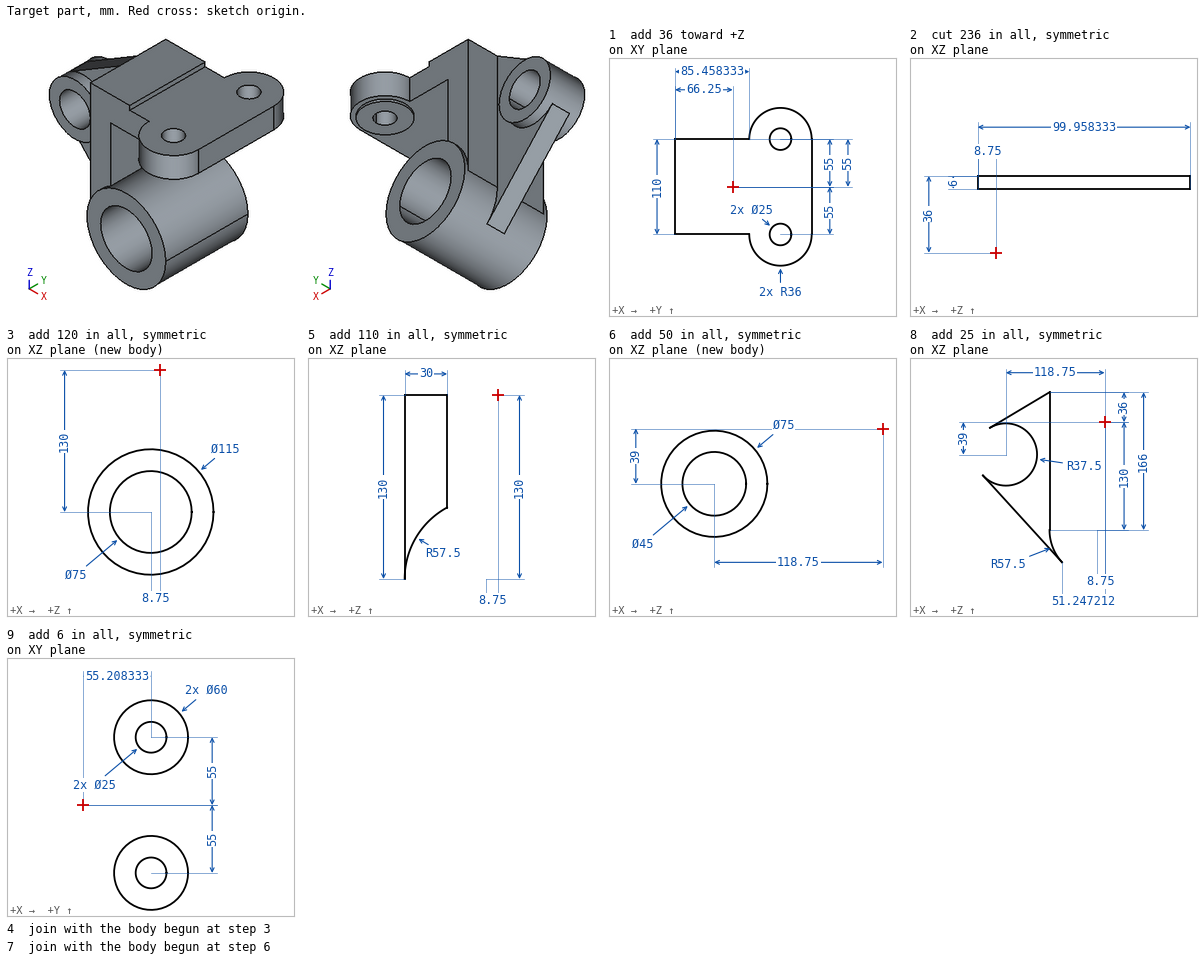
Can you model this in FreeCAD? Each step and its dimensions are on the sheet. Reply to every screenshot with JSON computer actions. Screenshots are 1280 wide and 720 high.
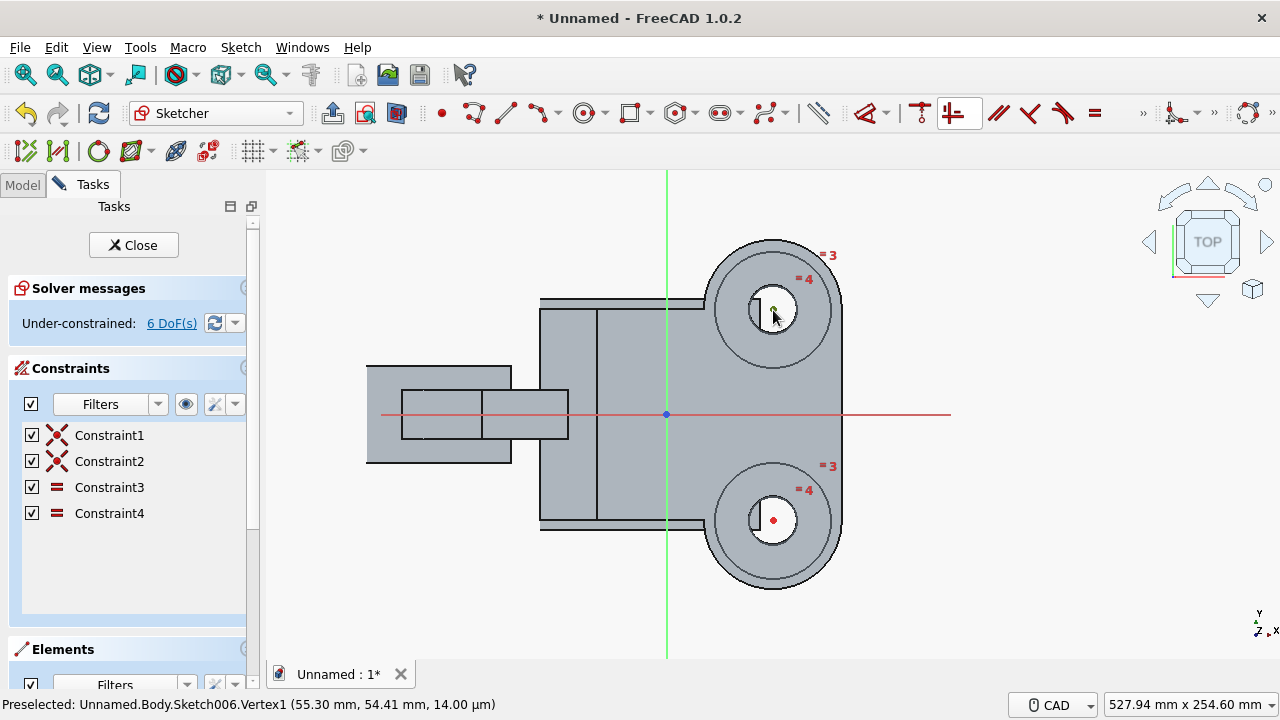
{"action": "left_click", "coordinate": [773, 521]}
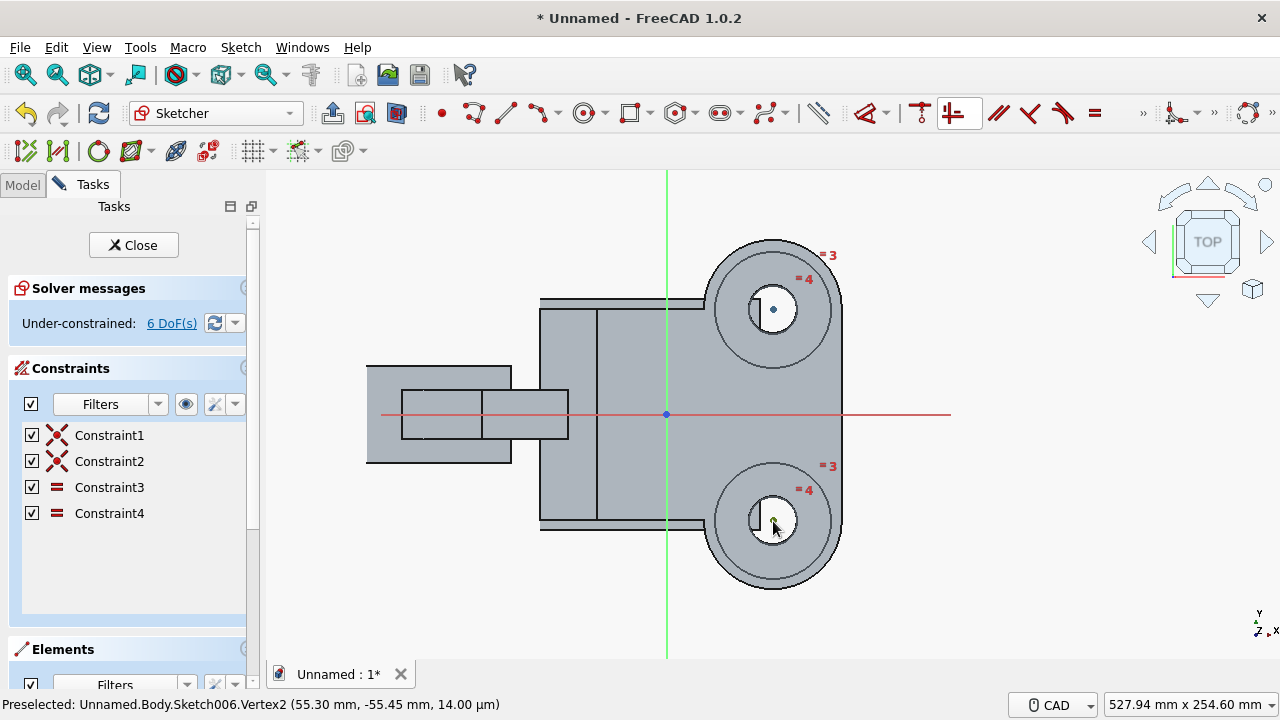
{"action": "key", "text": "v"}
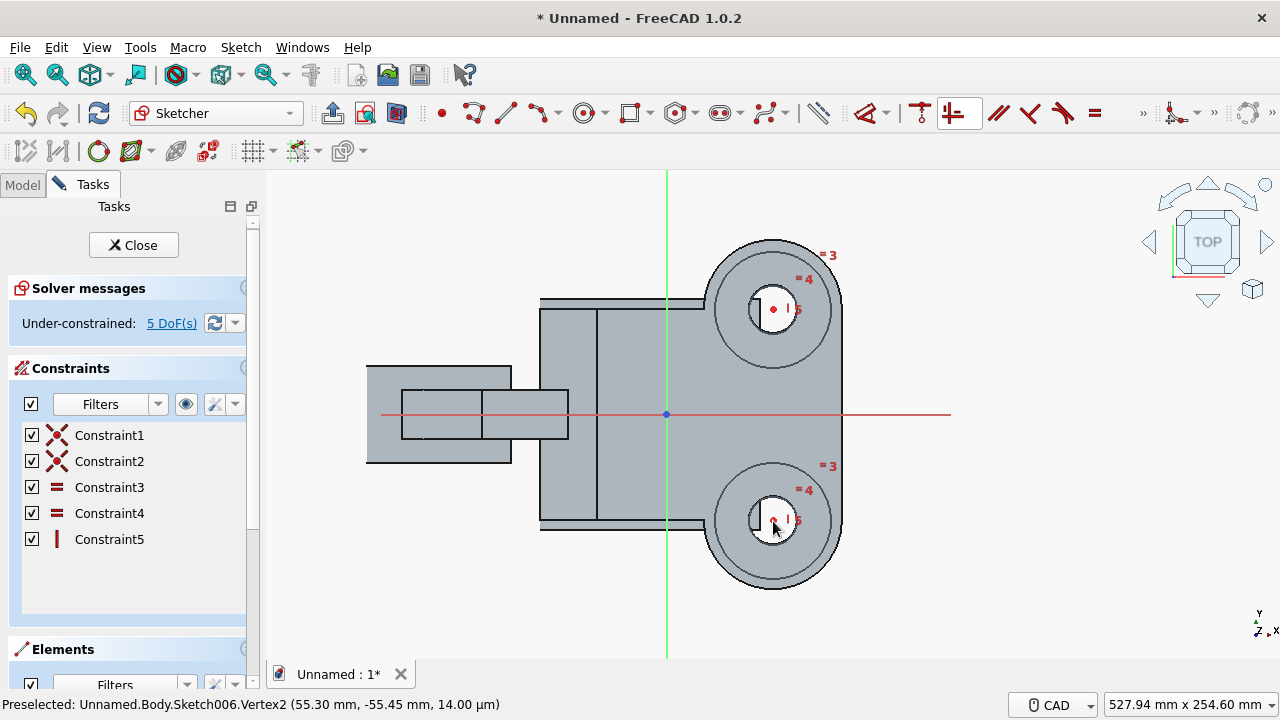
{"action": "left_click", "coordinate": [866, 114]}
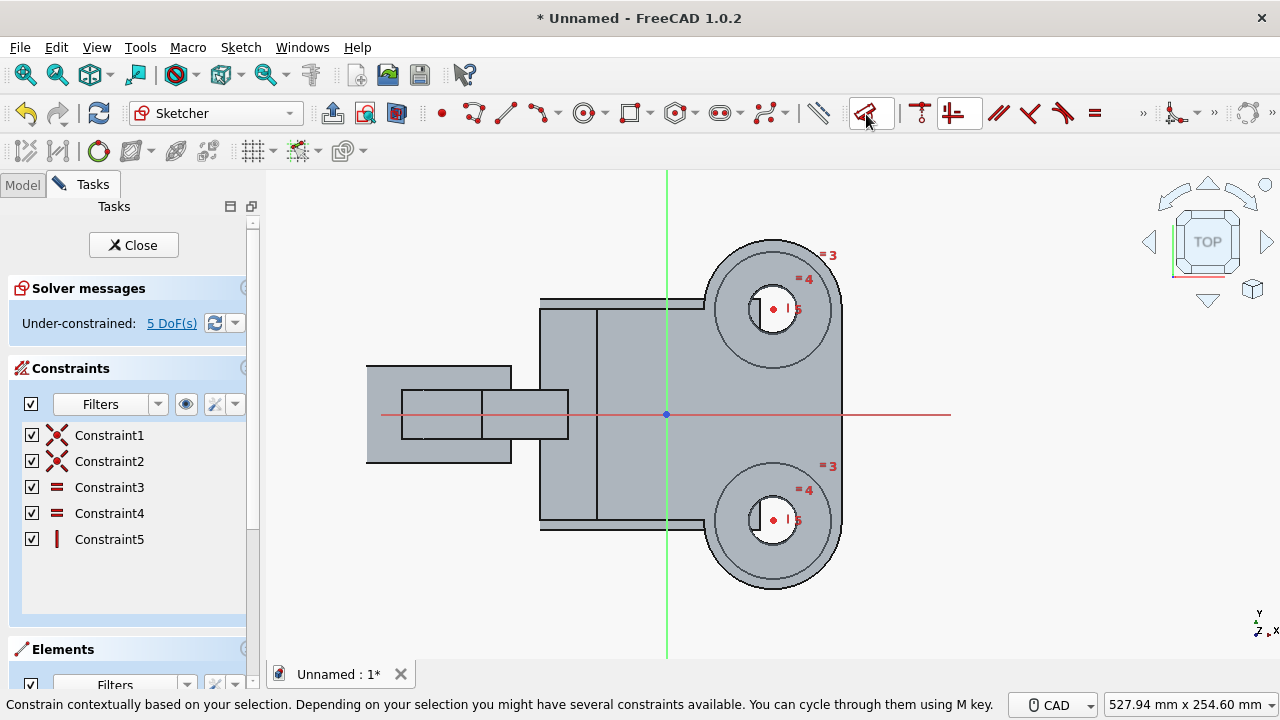
{"action": "left_click", "coordinate": [814, 269]}
{"action": "left_click", "coordinate": [837, 246]}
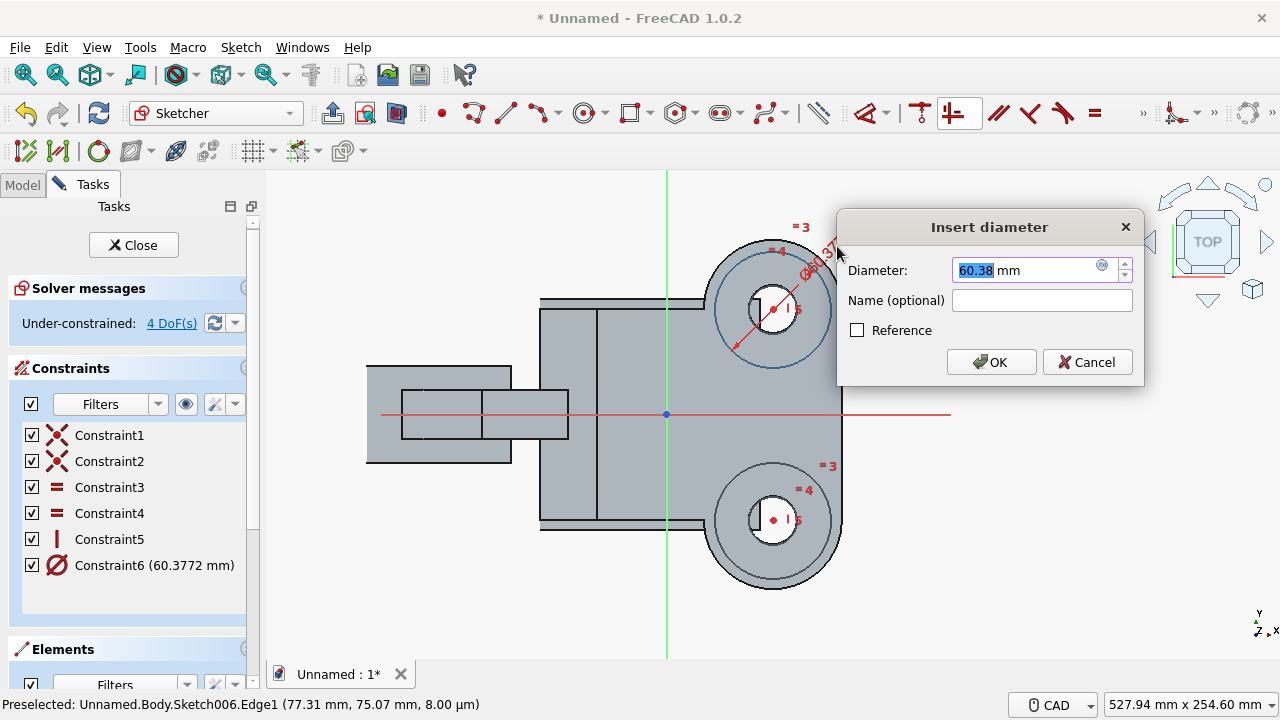
{"action": "type", "text": "60"}
{"action": "key", "text": "Return"}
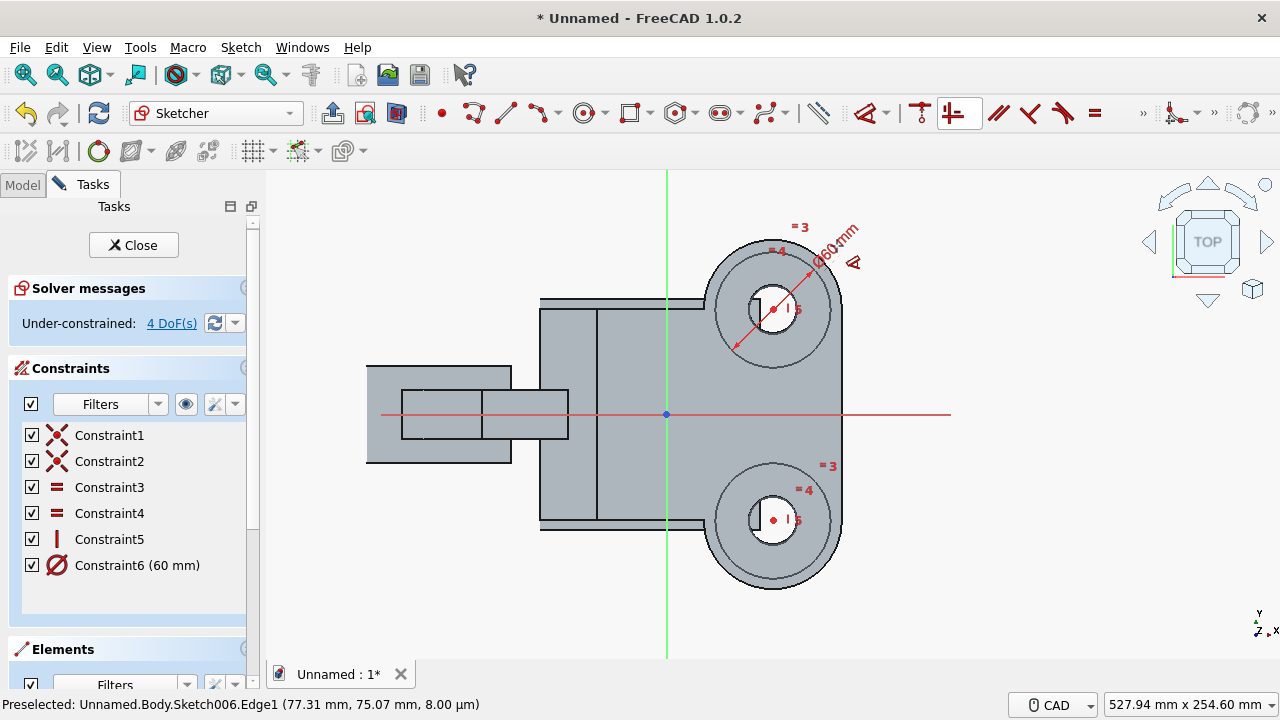
{"action": "left_click", "coordinate": [790, 293]}
{"action": "left_click", "coordinate": [849, 288]}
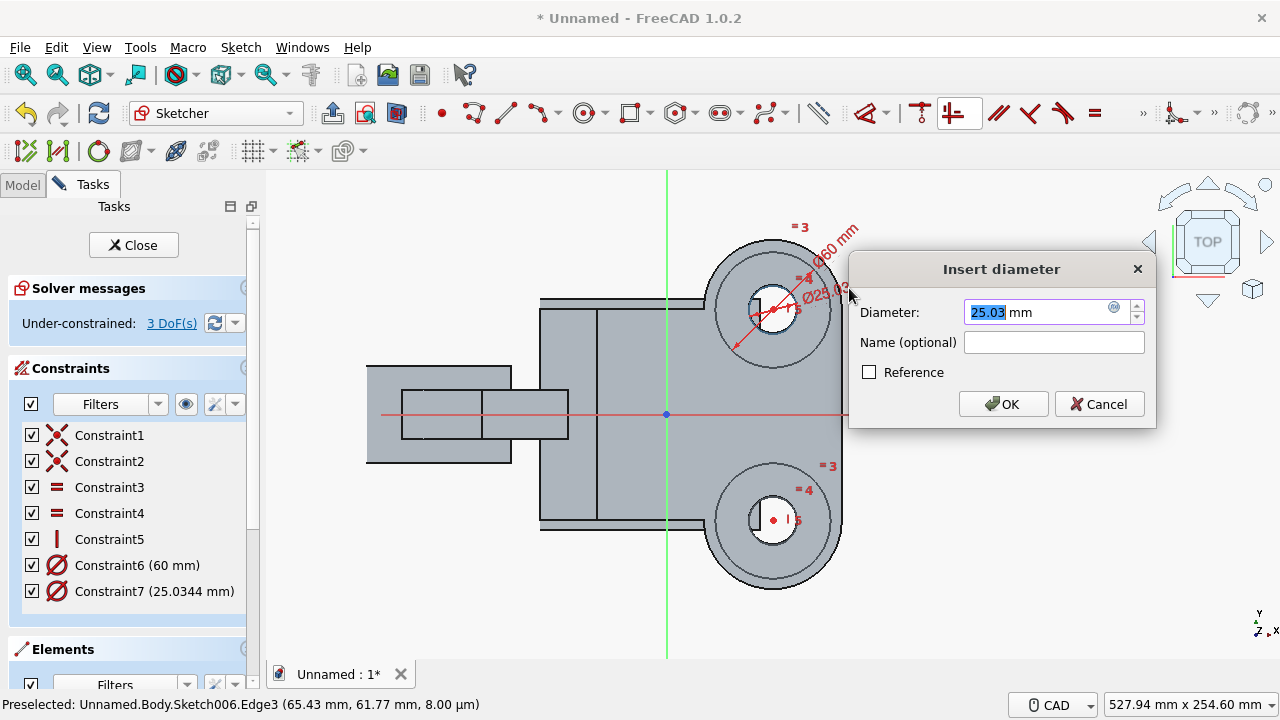
{"action": "type", "text": "25"}
{"action": "key", "text": "Return"}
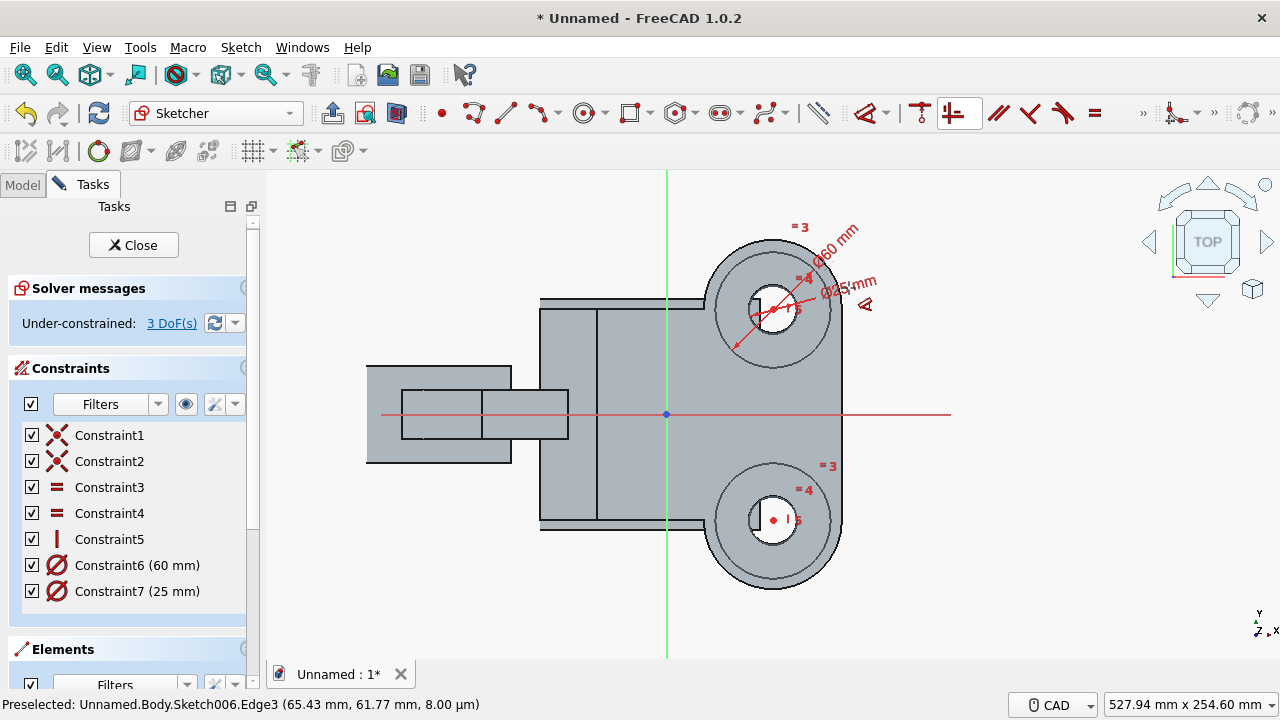
{"action": "left_click", "coordinate": [773, 310]}
{"action": "left_click", "coordinate": [633, 362]}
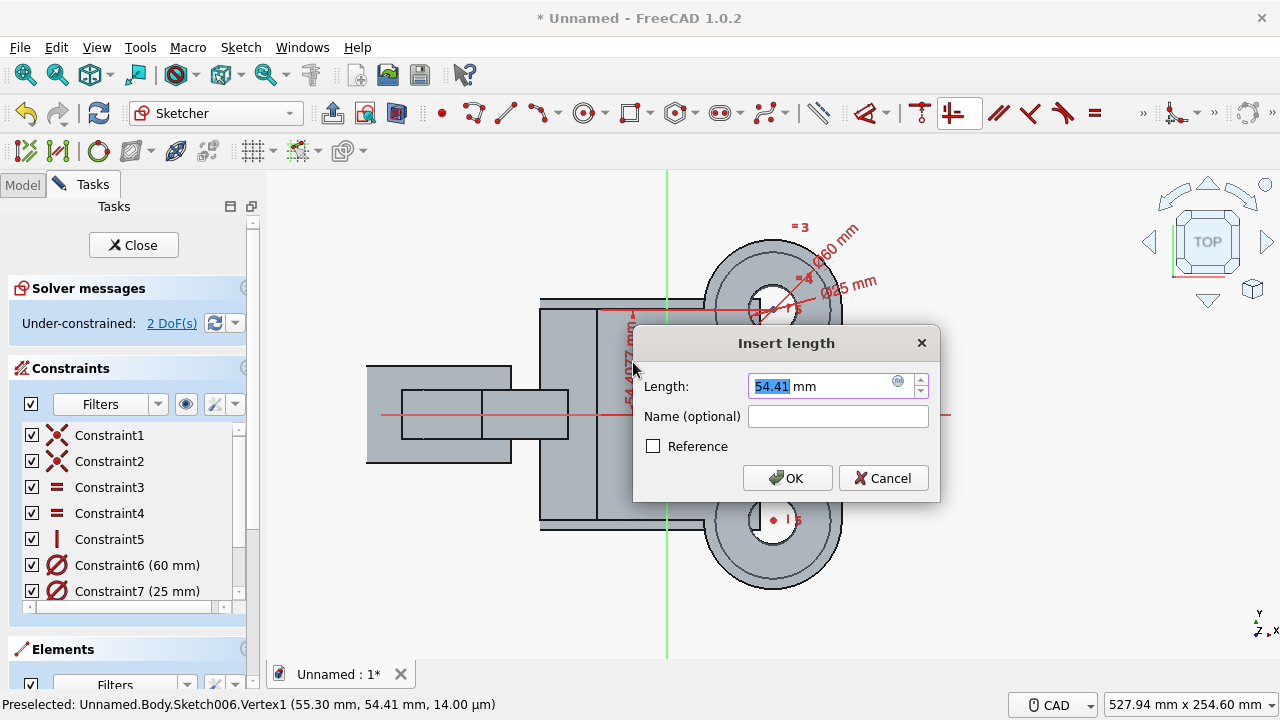
{"action": "type", "text": "55"}
{"action": "key", "text": "Return"}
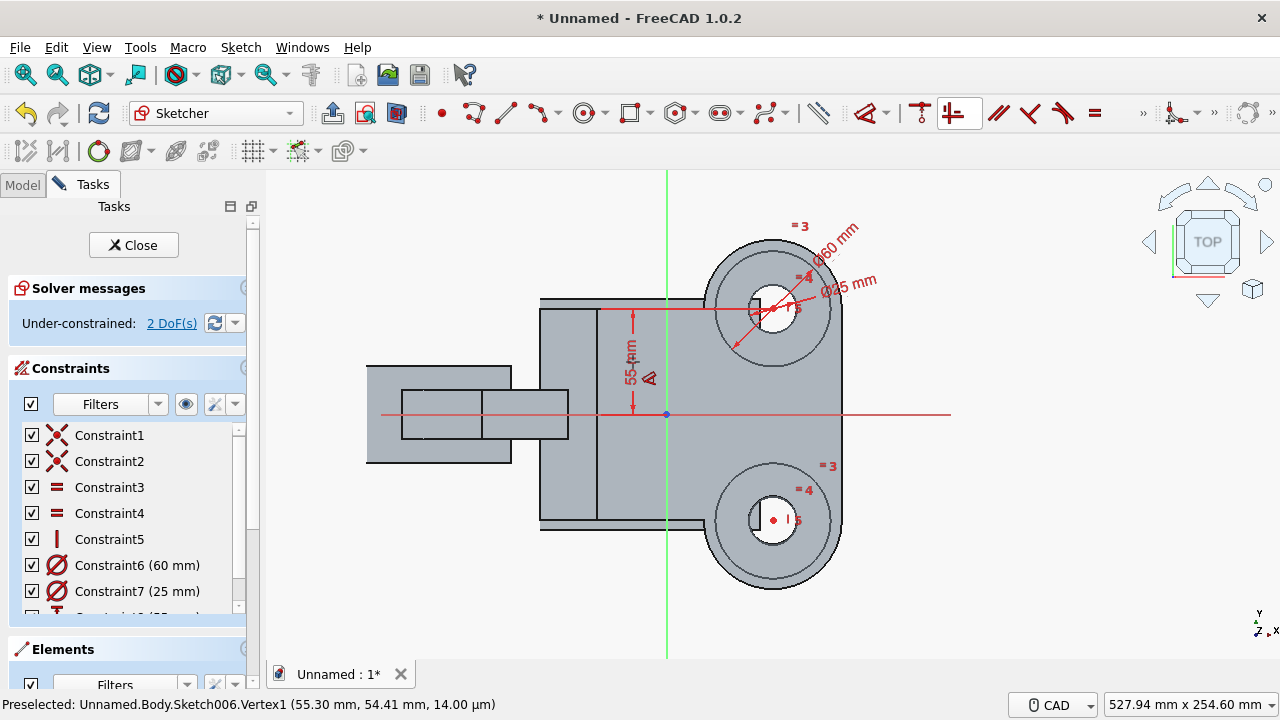
{"action": "left_click", "coordinate": [773, 521]}
{"action": "left_click", "coordinate": [633, 468]}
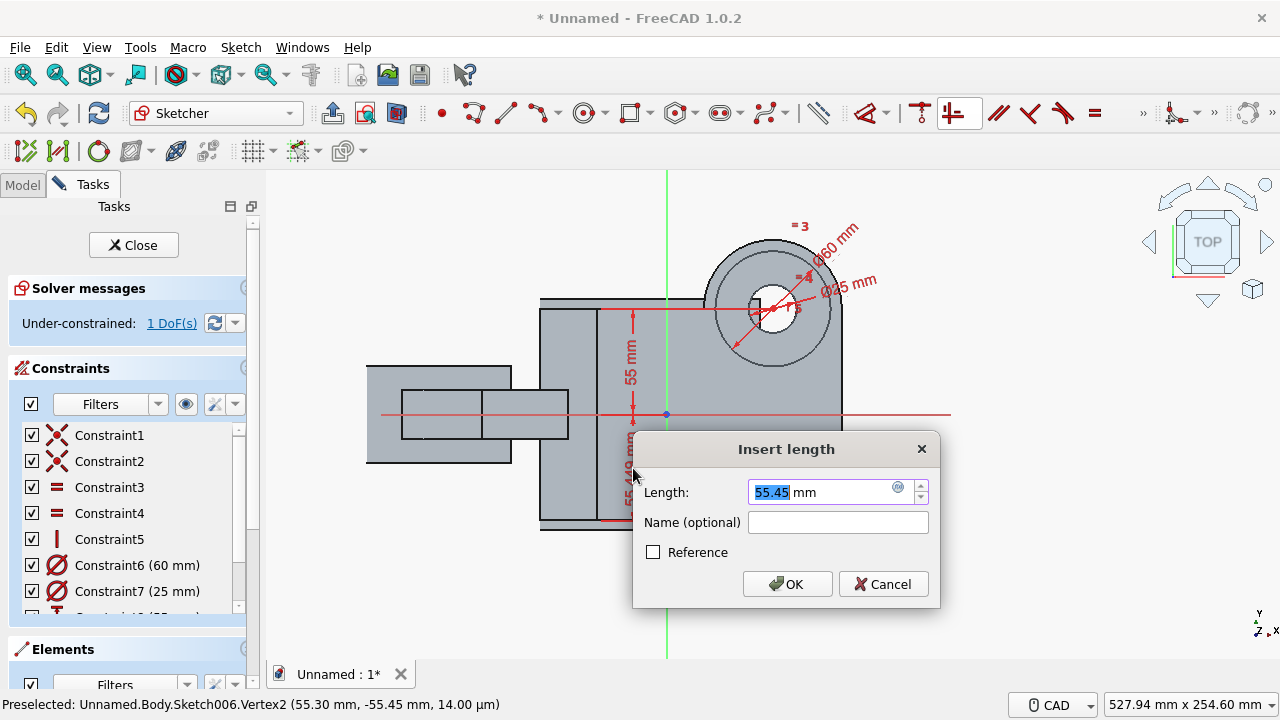
{"action": "type", "text": "55"}
{"action": "key", "text": "Return"}